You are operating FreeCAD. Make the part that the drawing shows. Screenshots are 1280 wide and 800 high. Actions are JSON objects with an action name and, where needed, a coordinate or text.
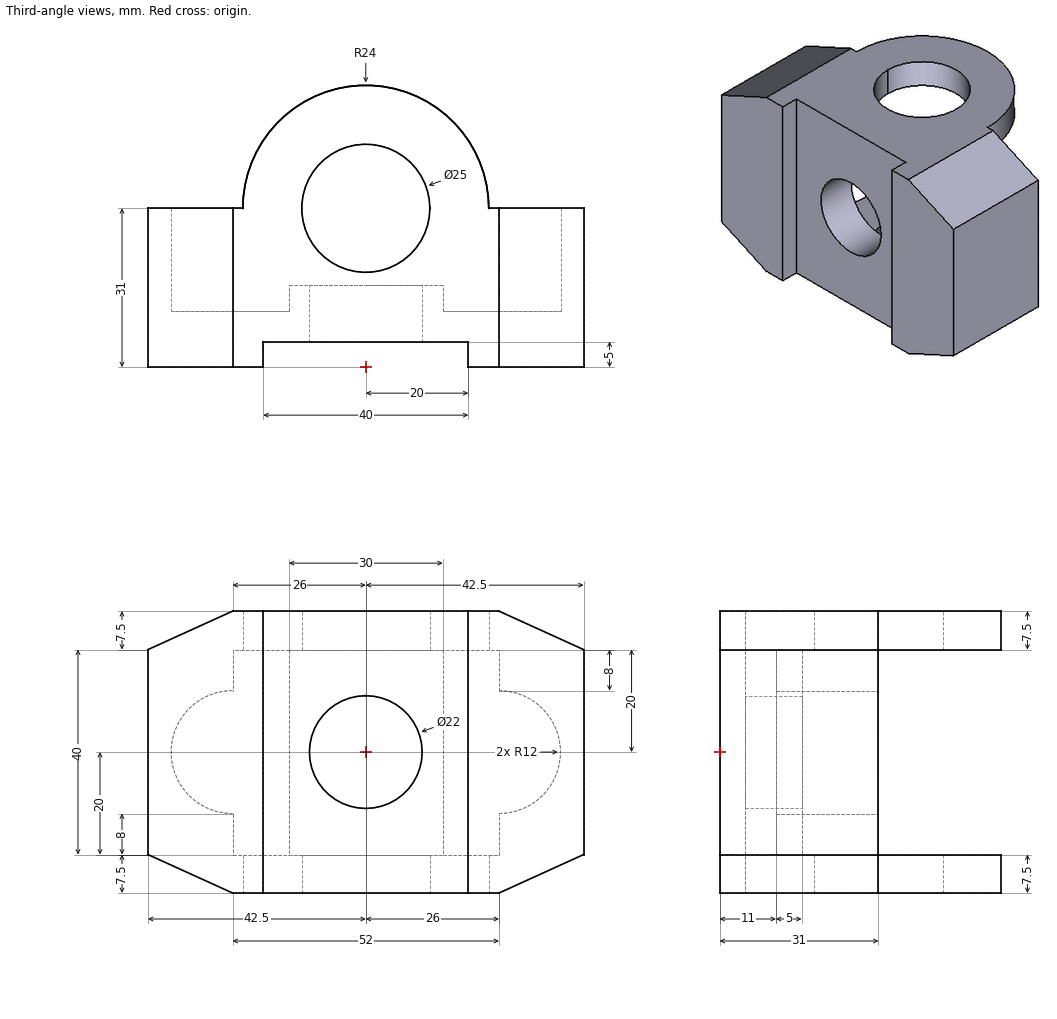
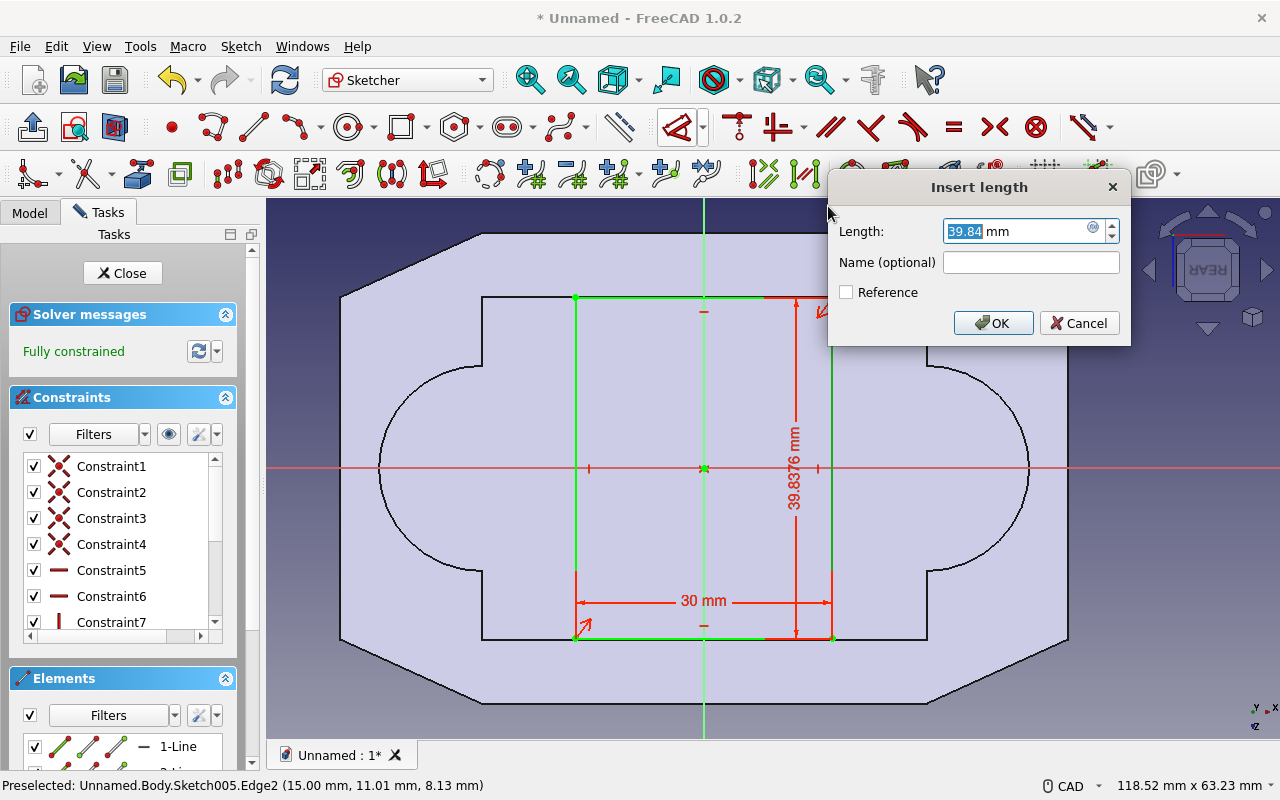
{"action": "type", "text": "40"}
{"action": "key", "text": "Return"}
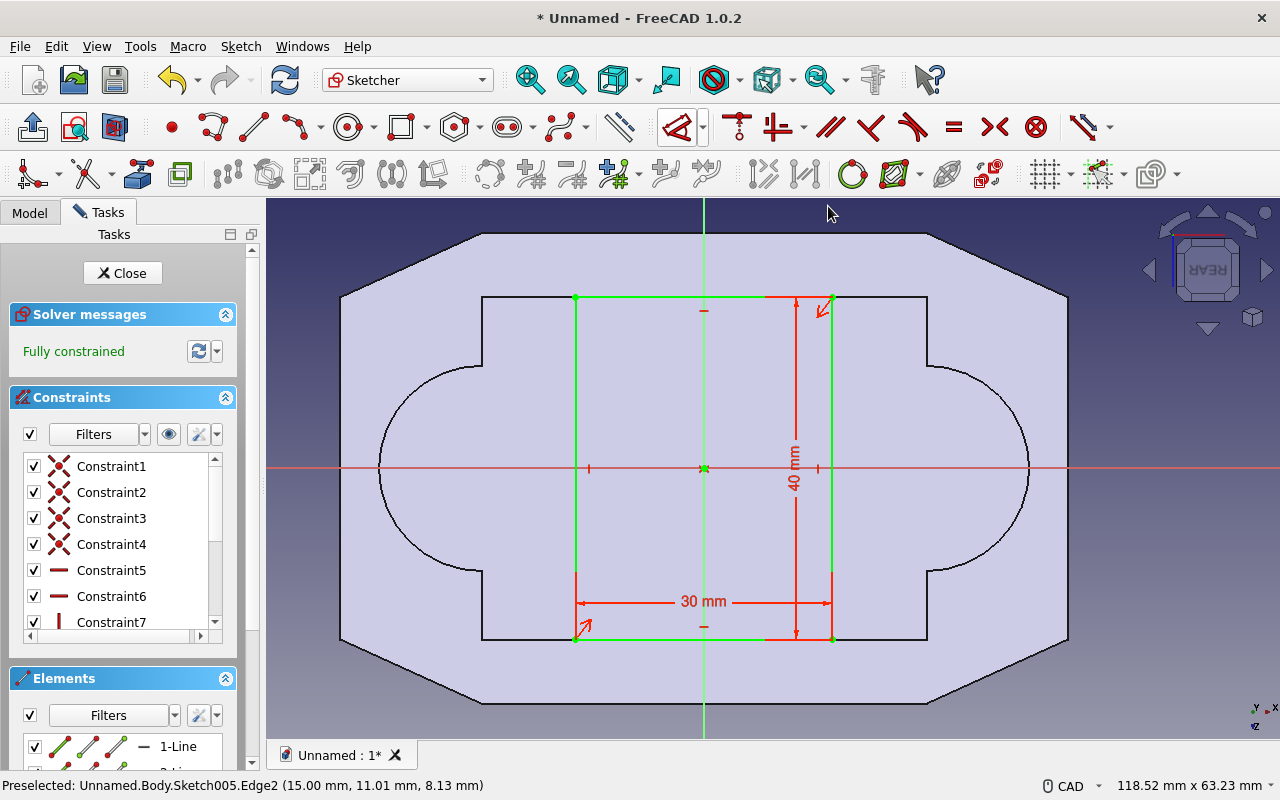
{"action": "left_click", "coordinate": [123, 273]}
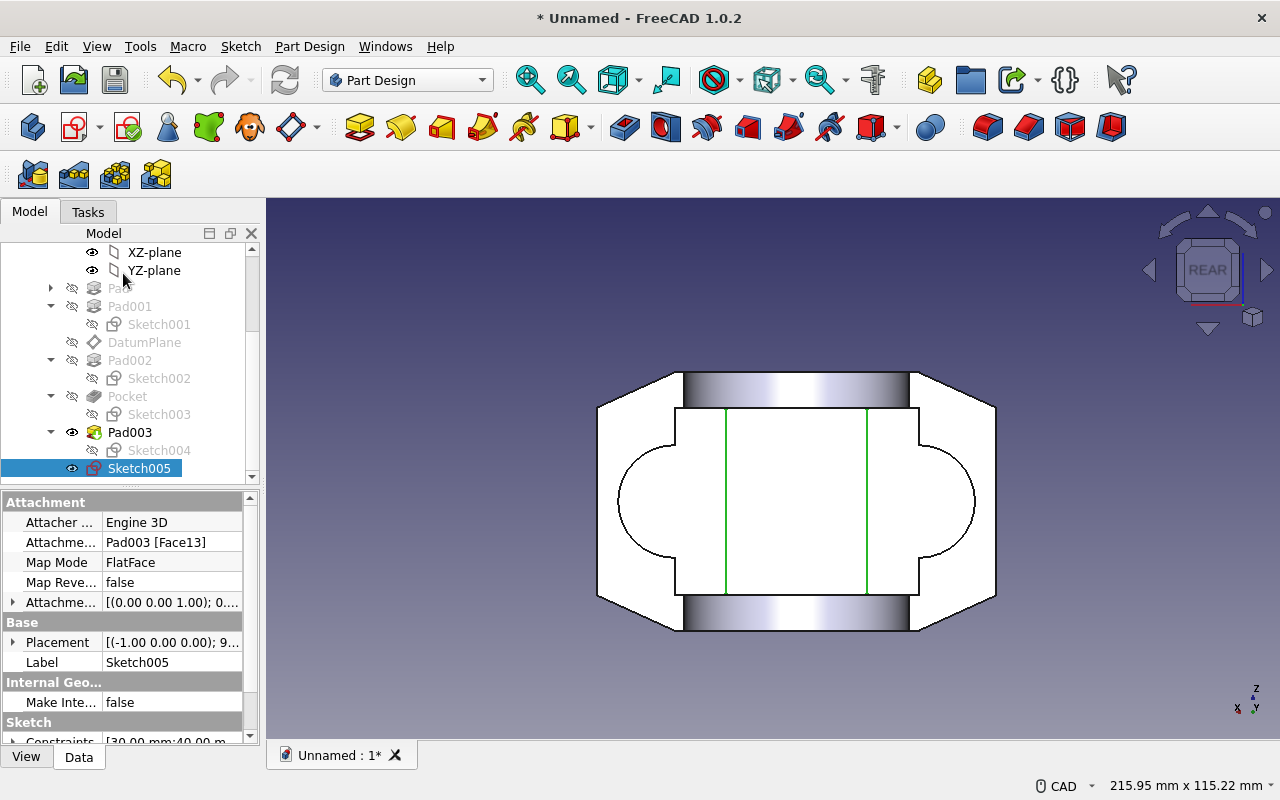
{"action": "left_click", "coordinate": [360, 128]}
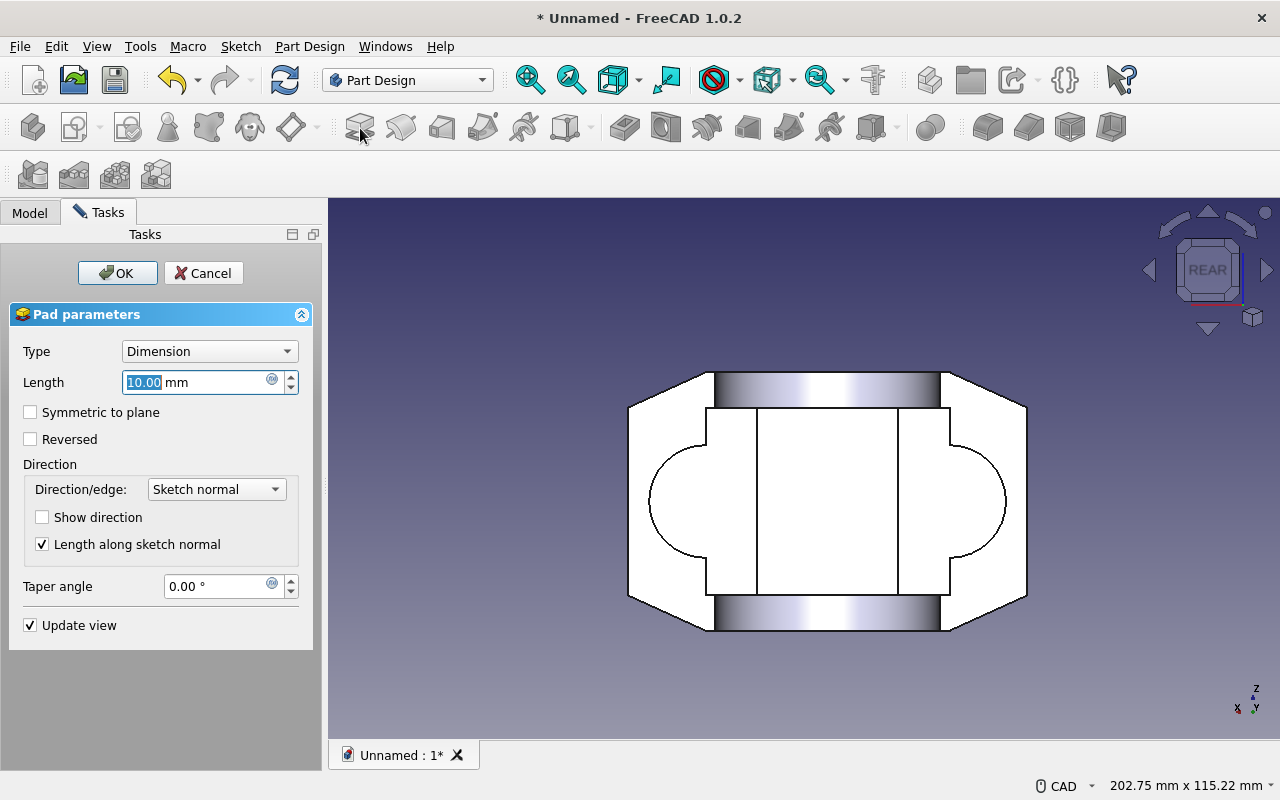
{"action": "type", "text": "5"}
{"action": "key", "text": "Tab"}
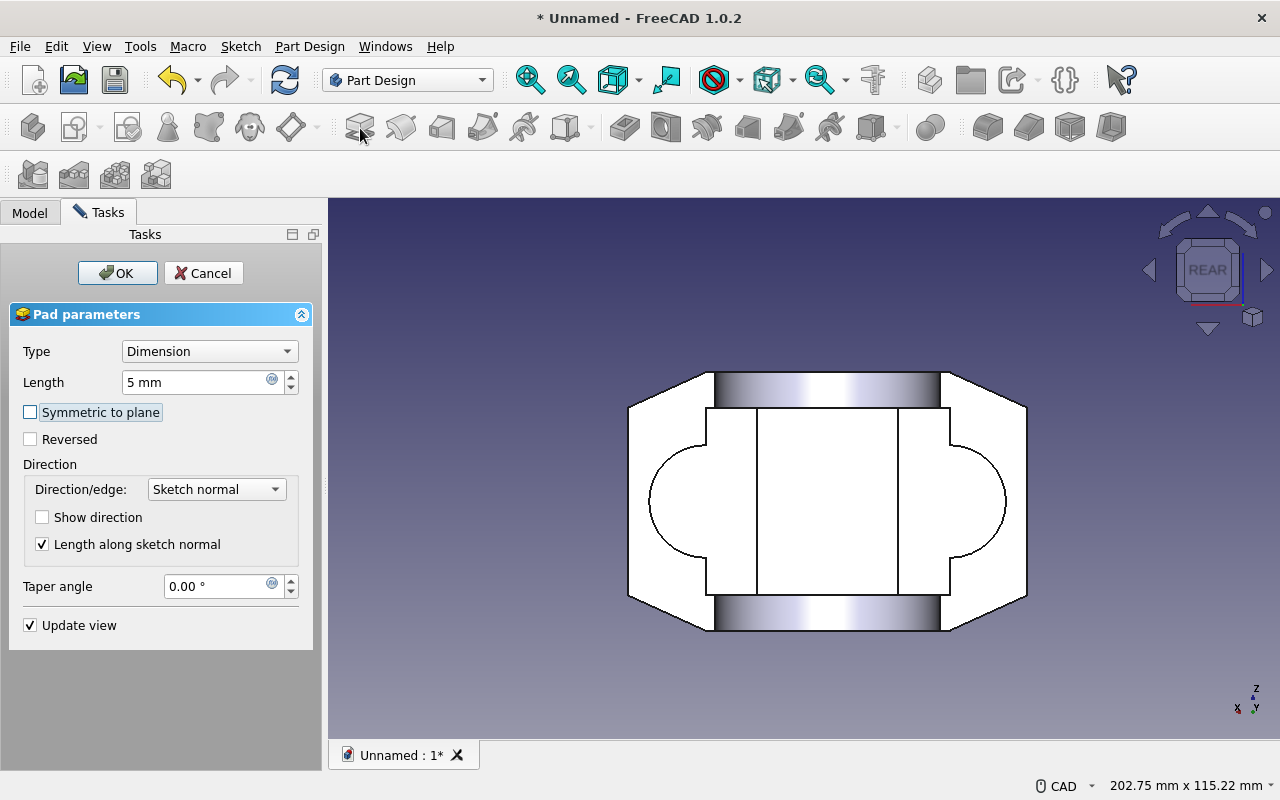
{"action": "left_click", "coordinate": [118, 273]}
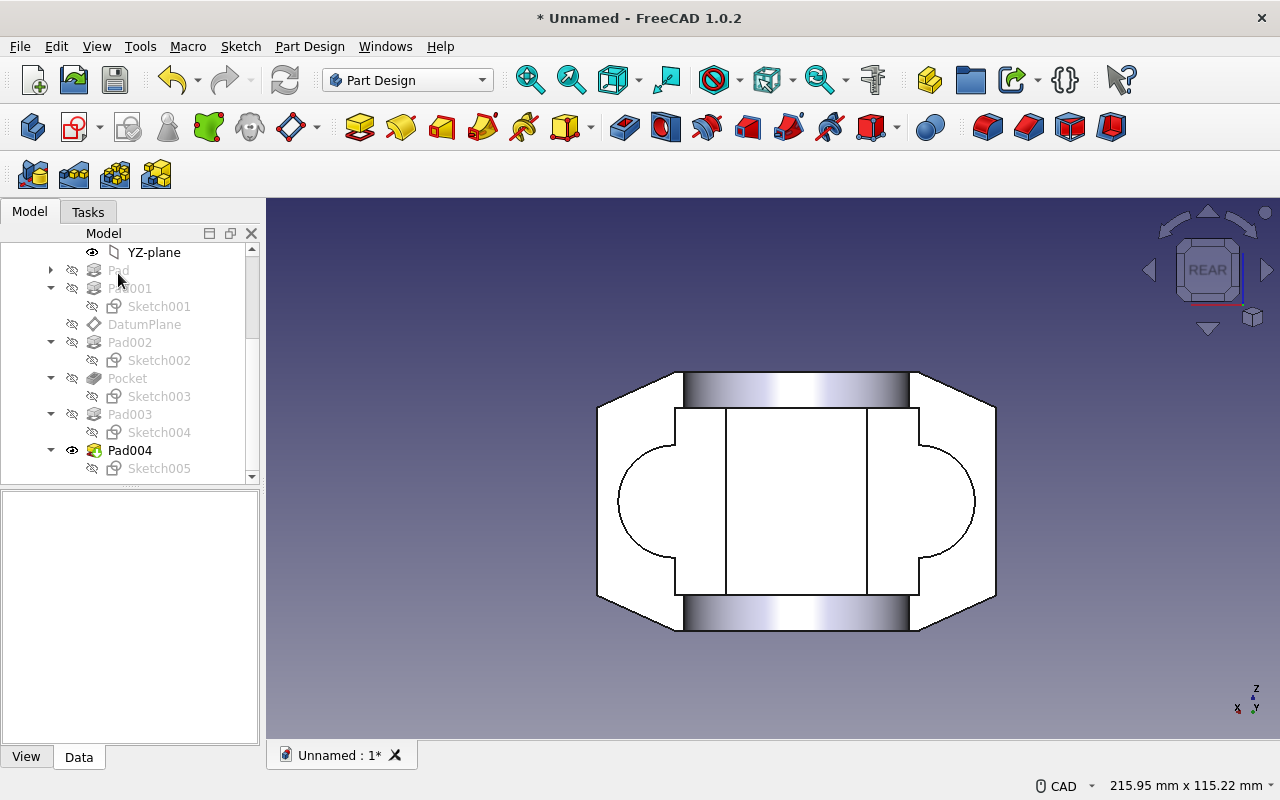
{"action": "left_click", "coordinate": [797, 501]}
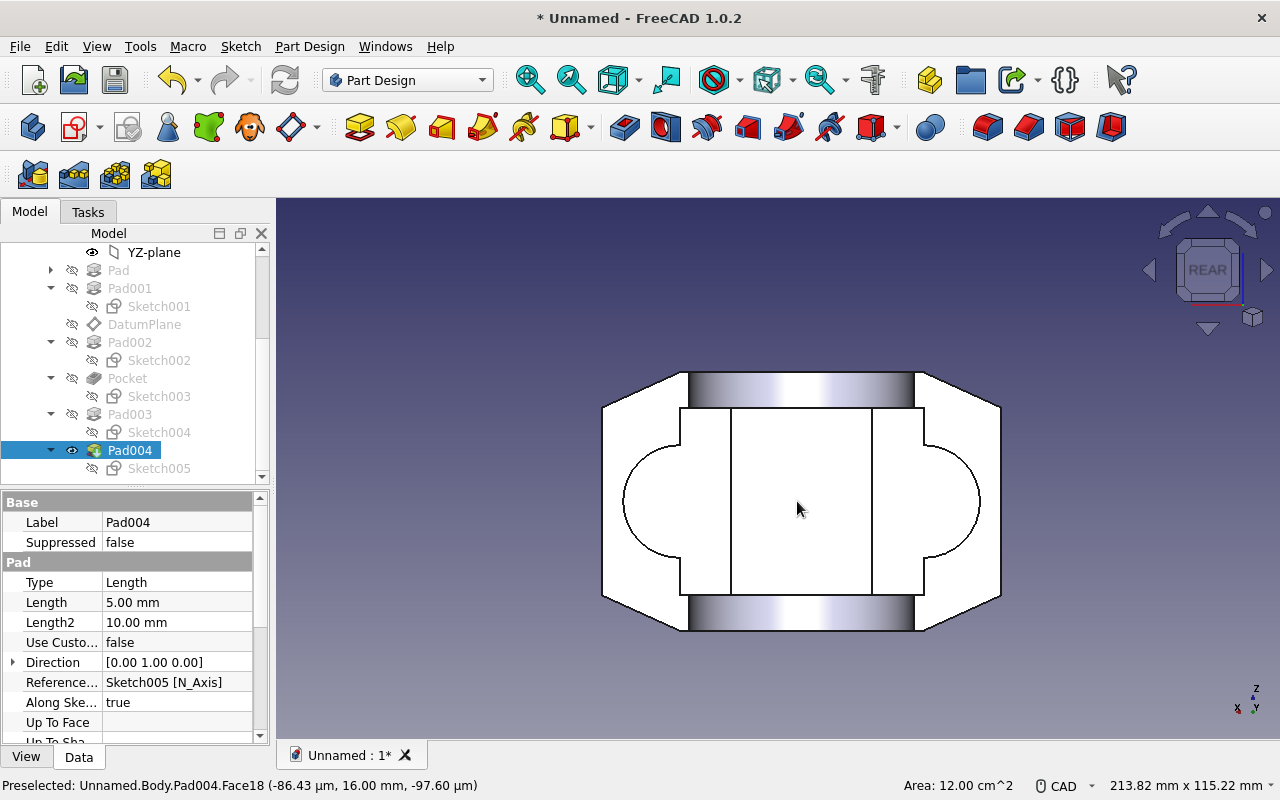
{"action": "left_click", "coordinate": [74, 128]}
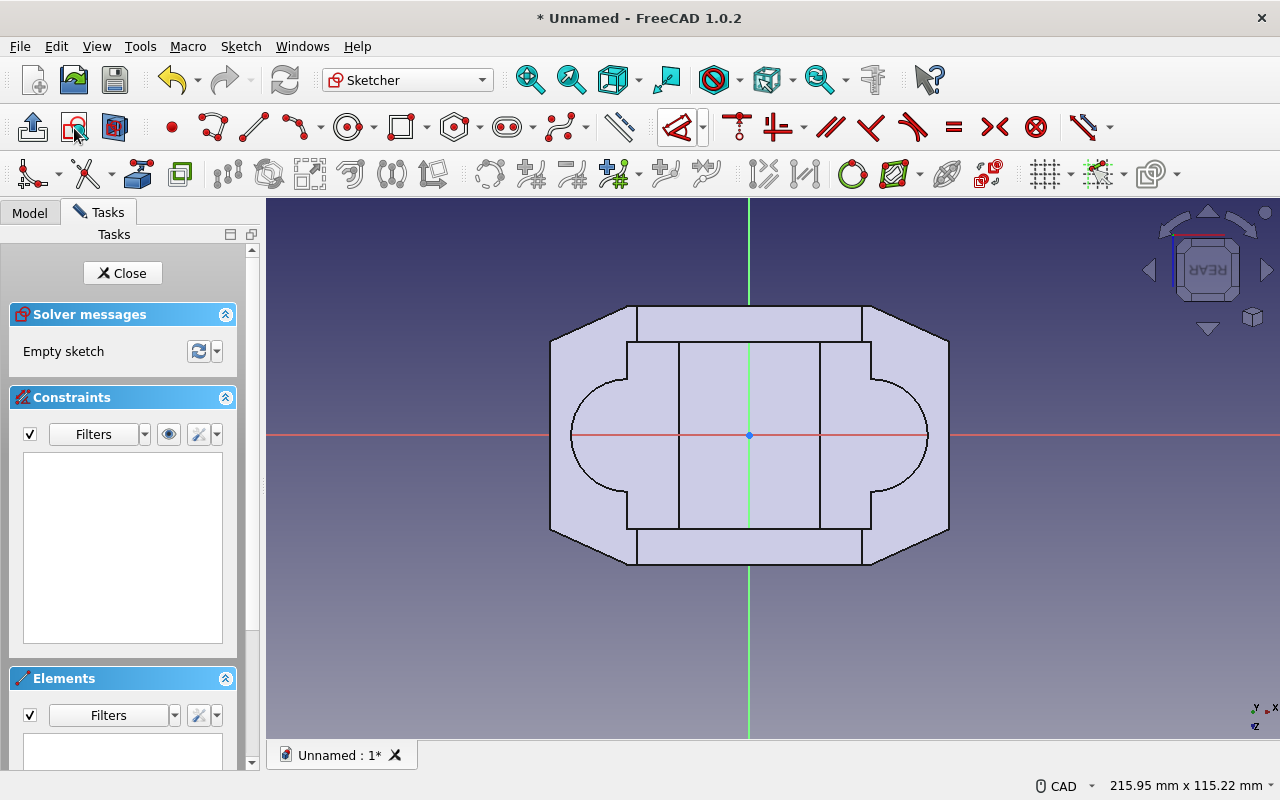
{"action": "scroll", "coordinate": [769, 421], "scroll_direction": "up", "scroll_amount": 6}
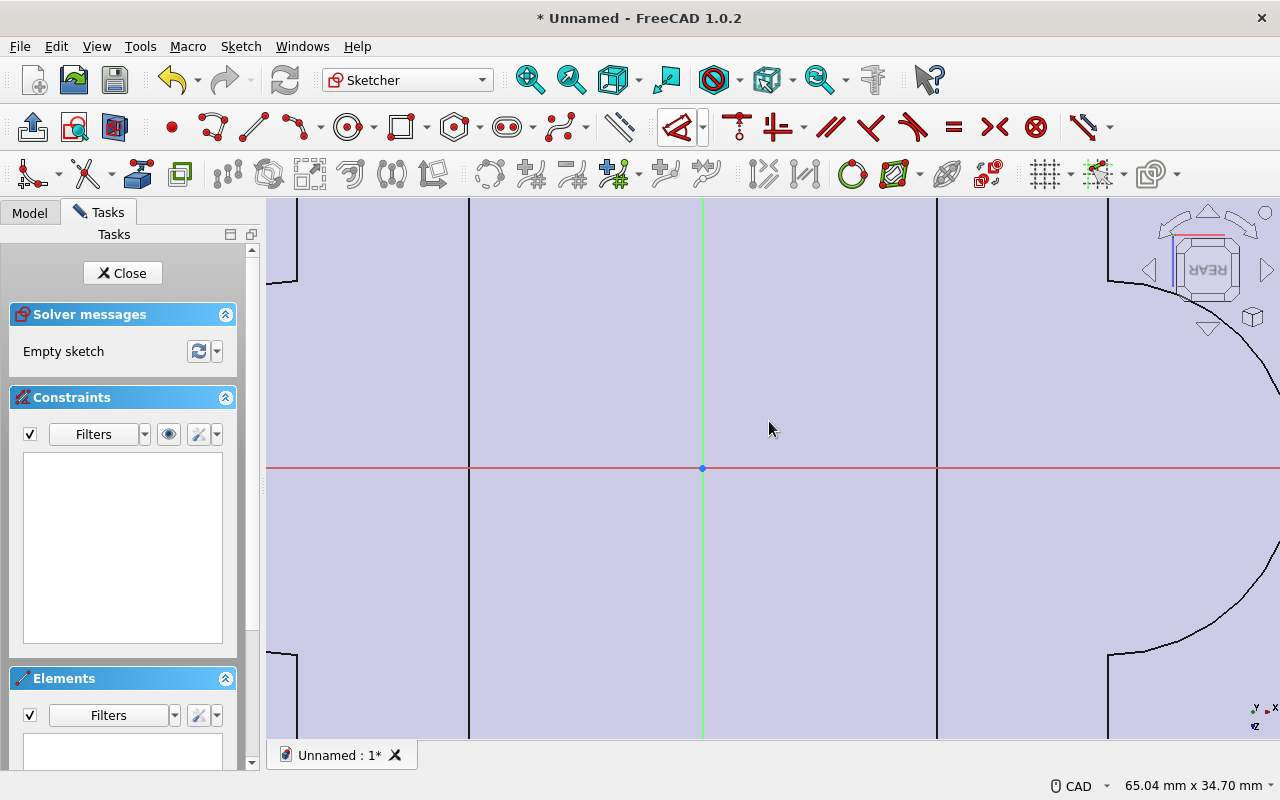
{"action": "left_click", "coordinate": [348, 128]}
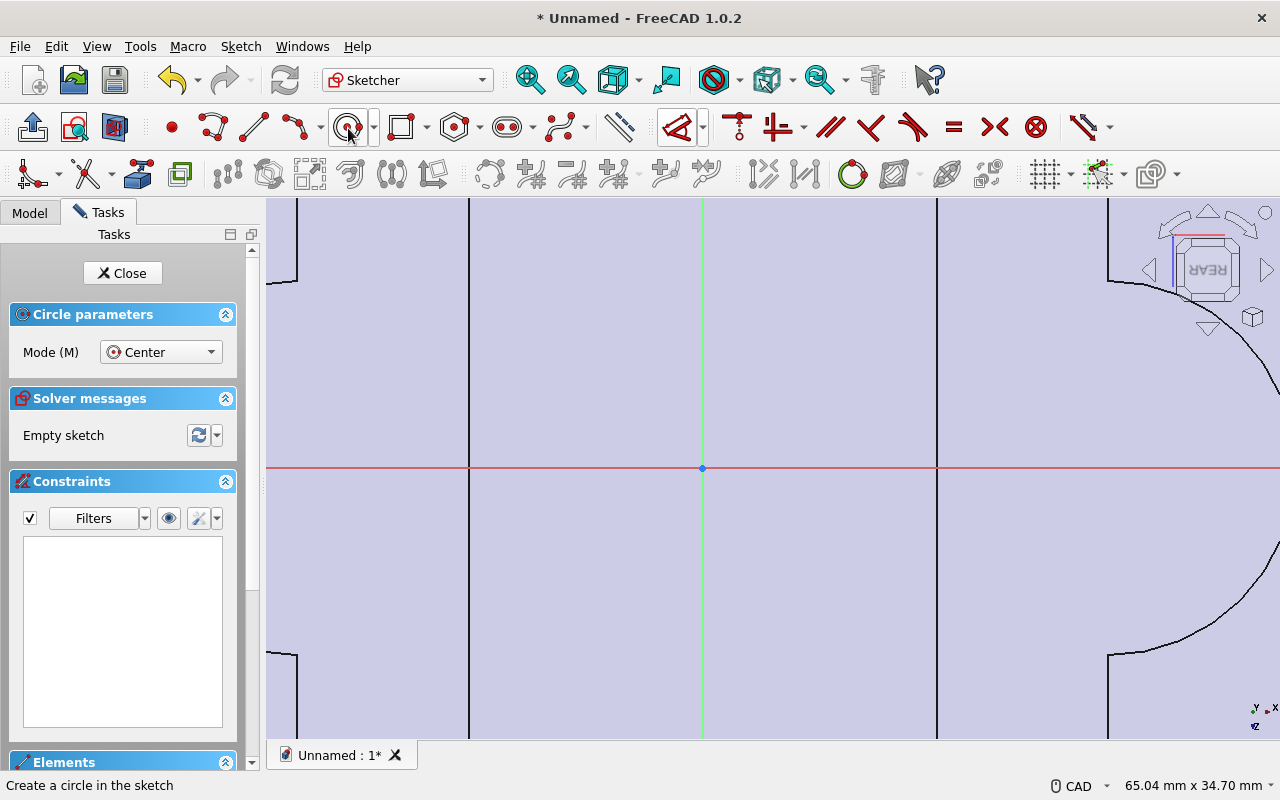
{"action": "left_click", "coordinate": [703, 468]}
{"action": "left_click", "coordinate": [824, 347]}
{"action": "key", "text": "Escape"}